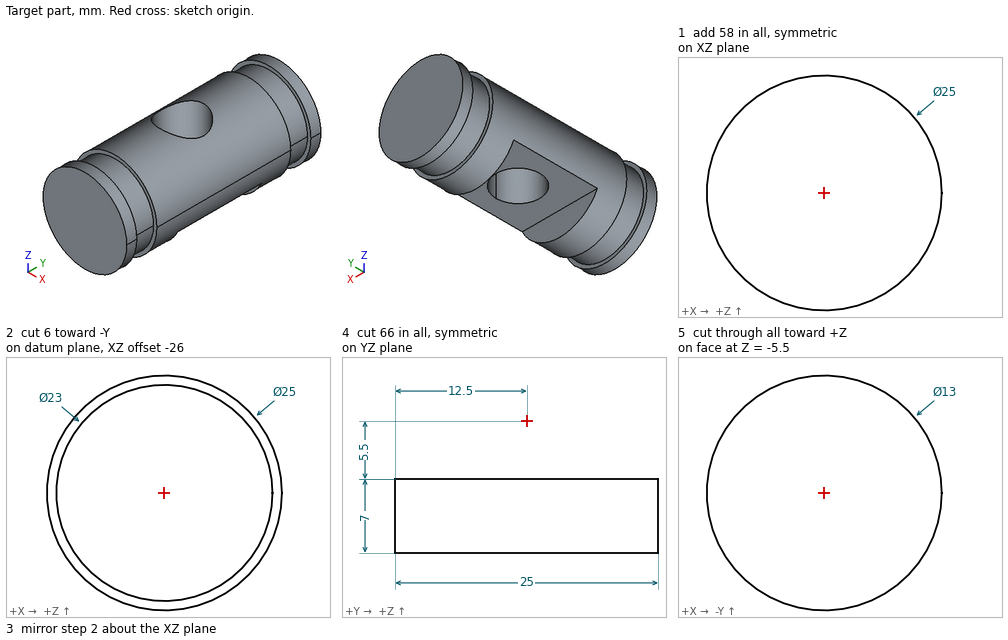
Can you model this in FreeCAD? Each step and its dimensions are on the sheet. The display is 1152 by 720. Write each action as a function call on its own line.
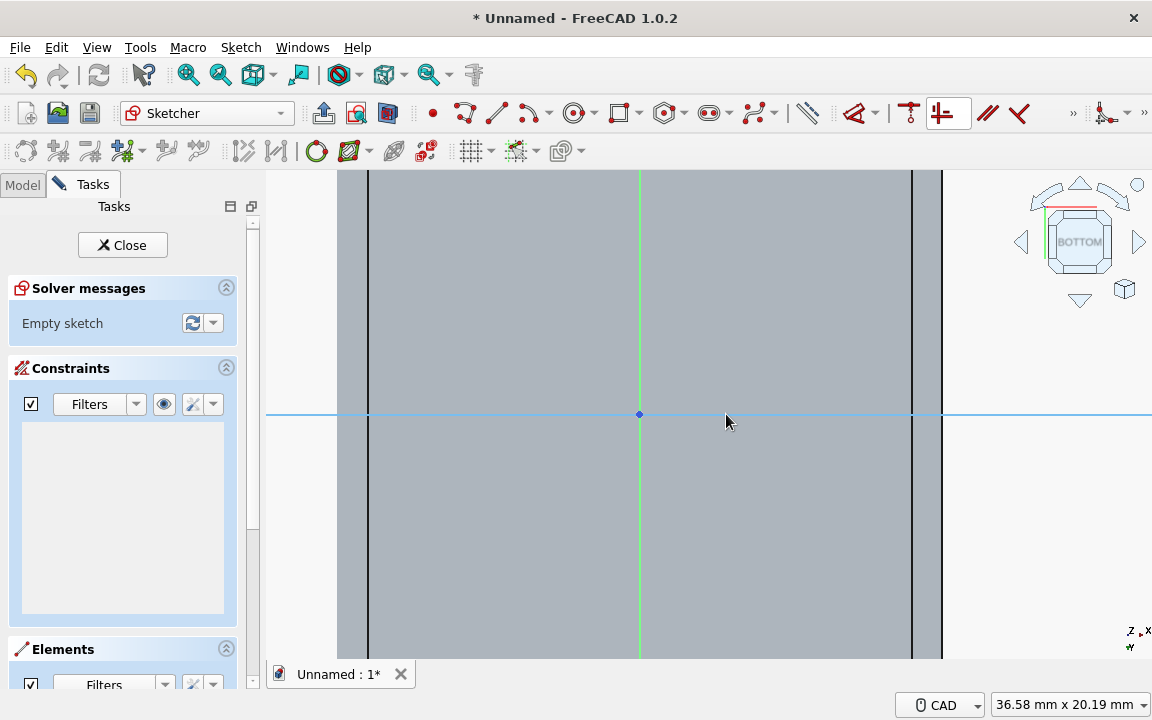
click(574, 114)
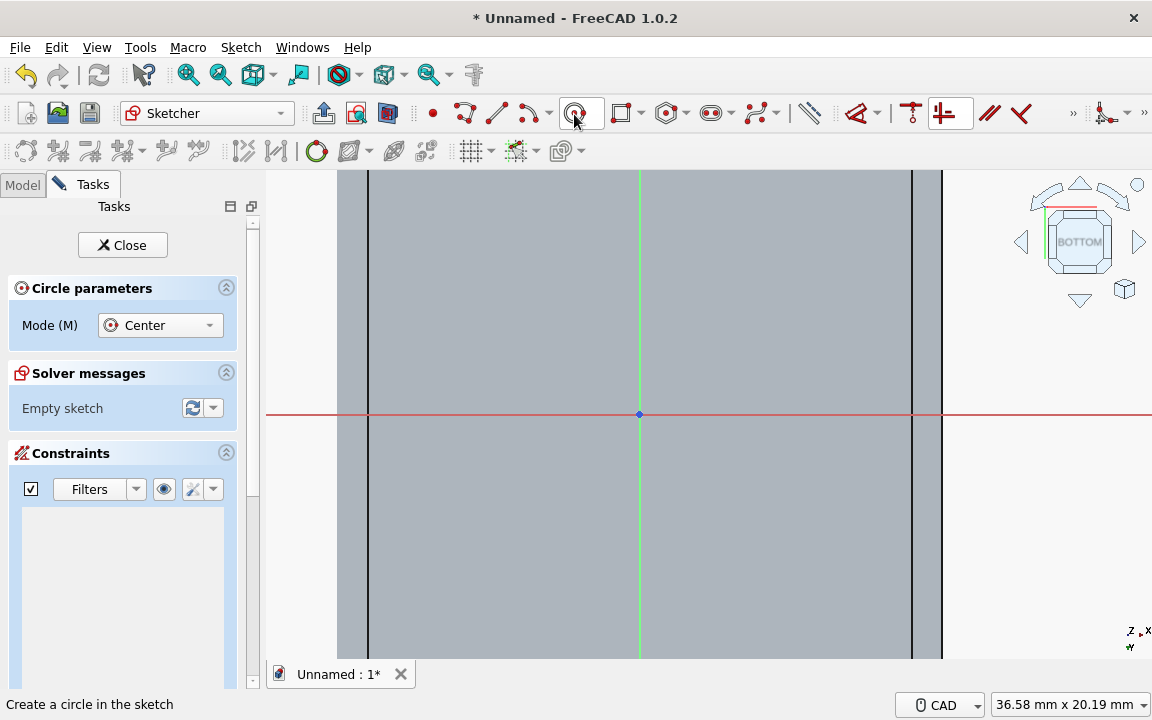
click(640, 414)
click(751, 303)
key(Escape)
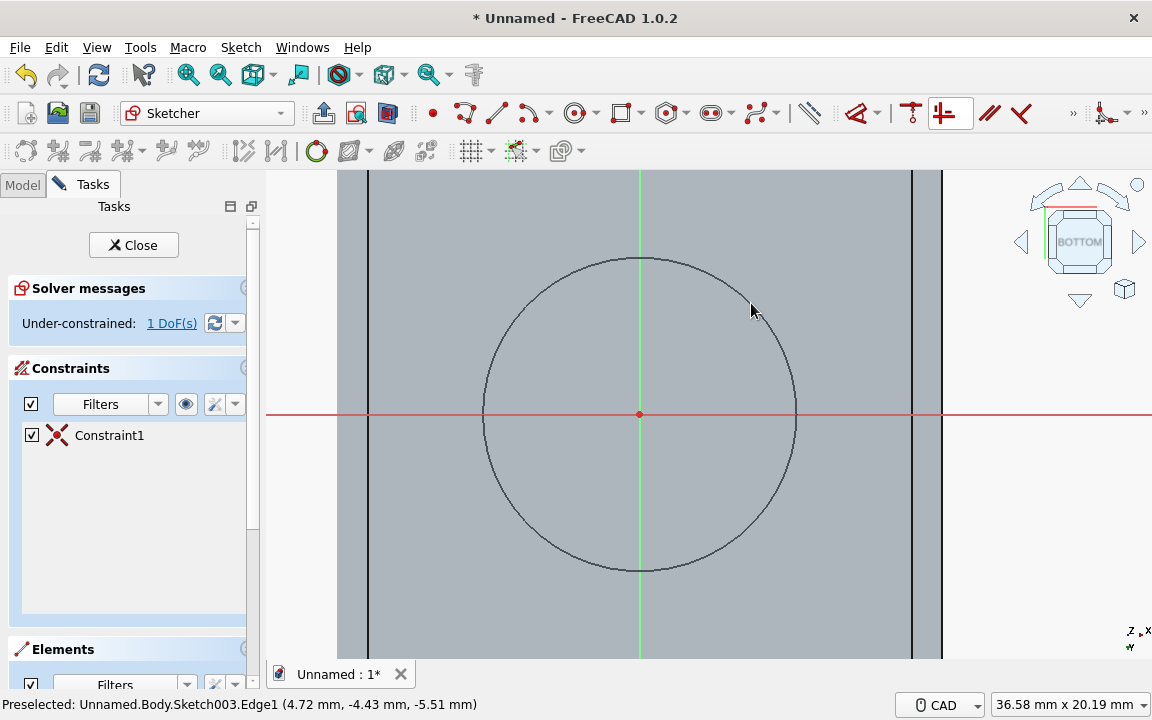
click(856, 114)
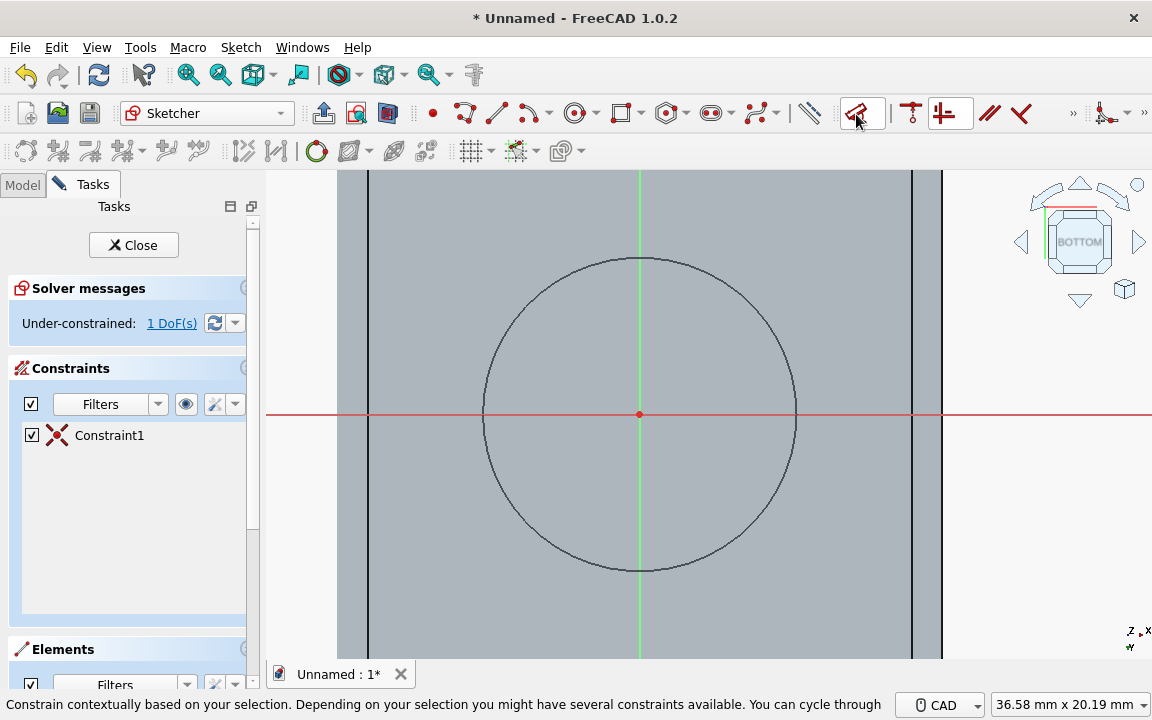
click(750, 303)
click(773, 280)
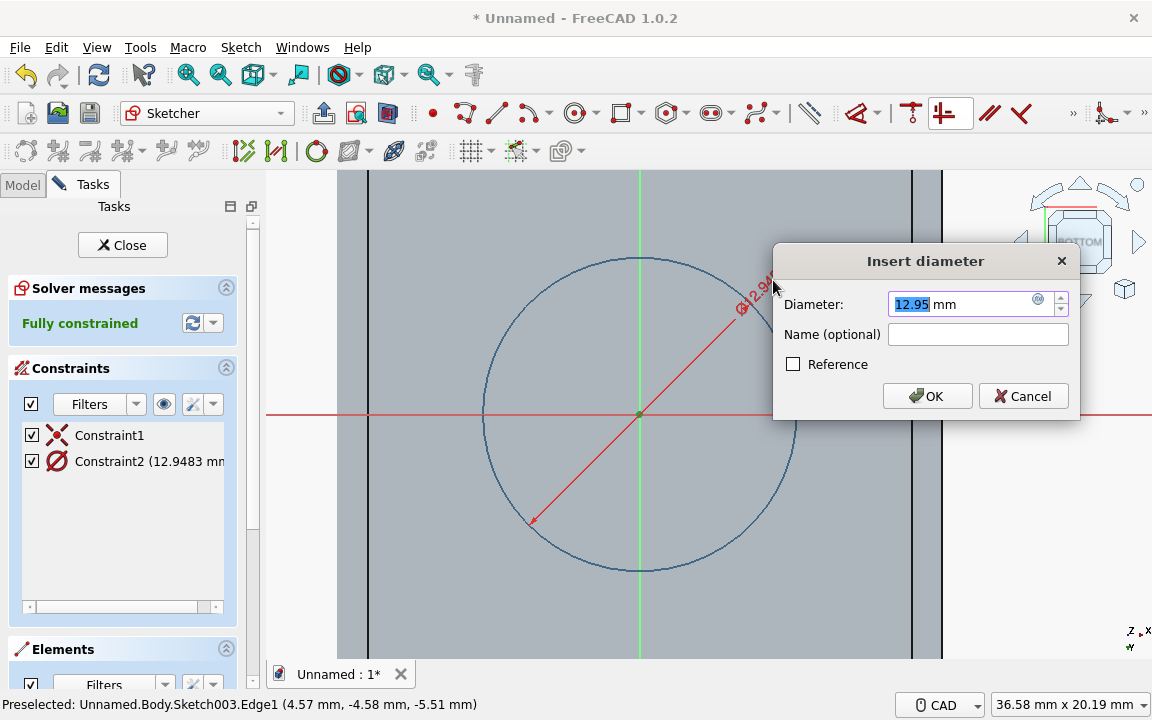
text(13)
key(Return)
key(Escape)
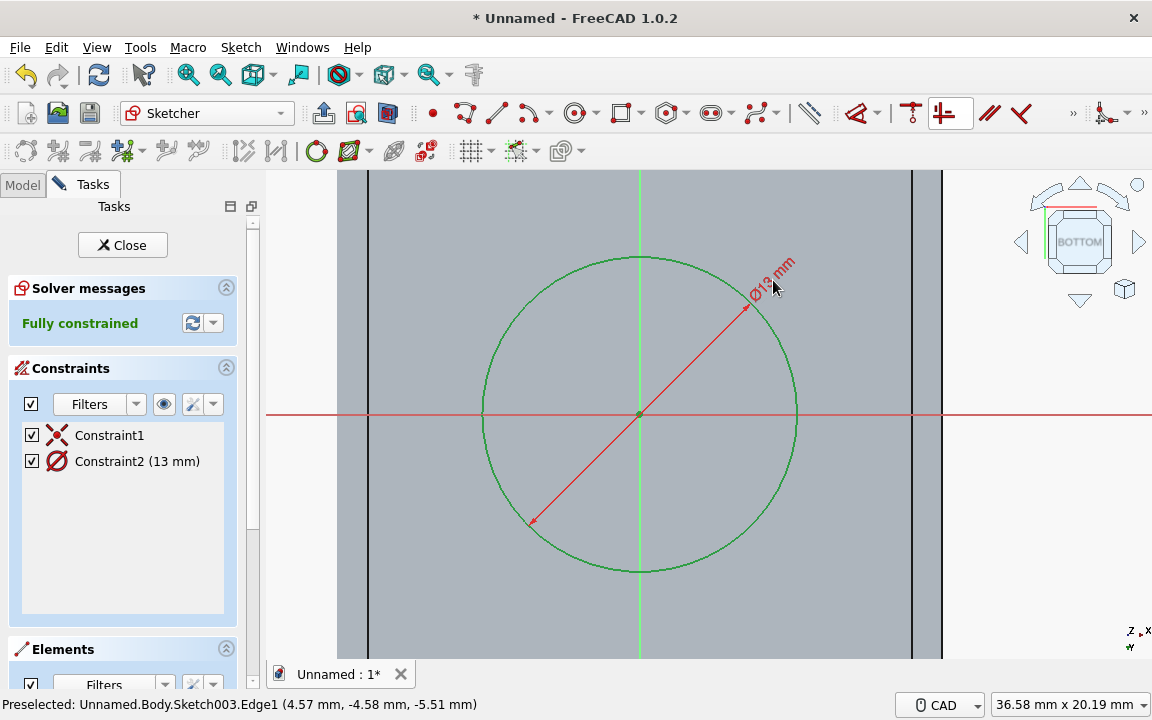
click(123, 245)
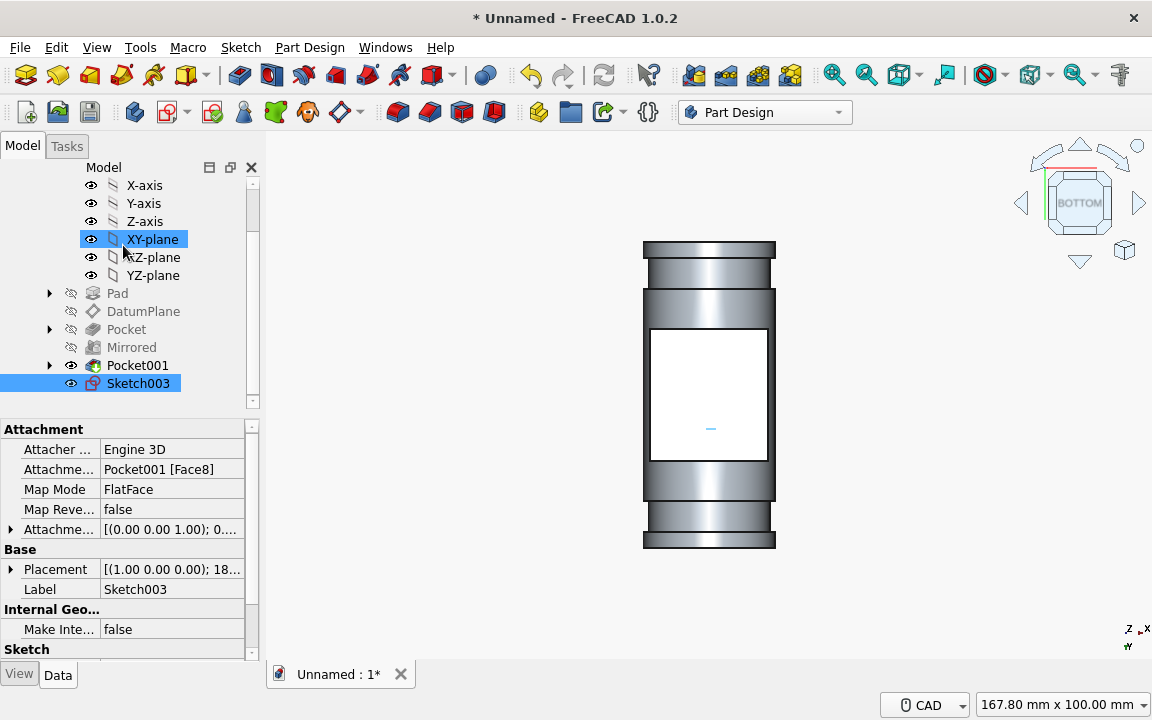
click(240, 76)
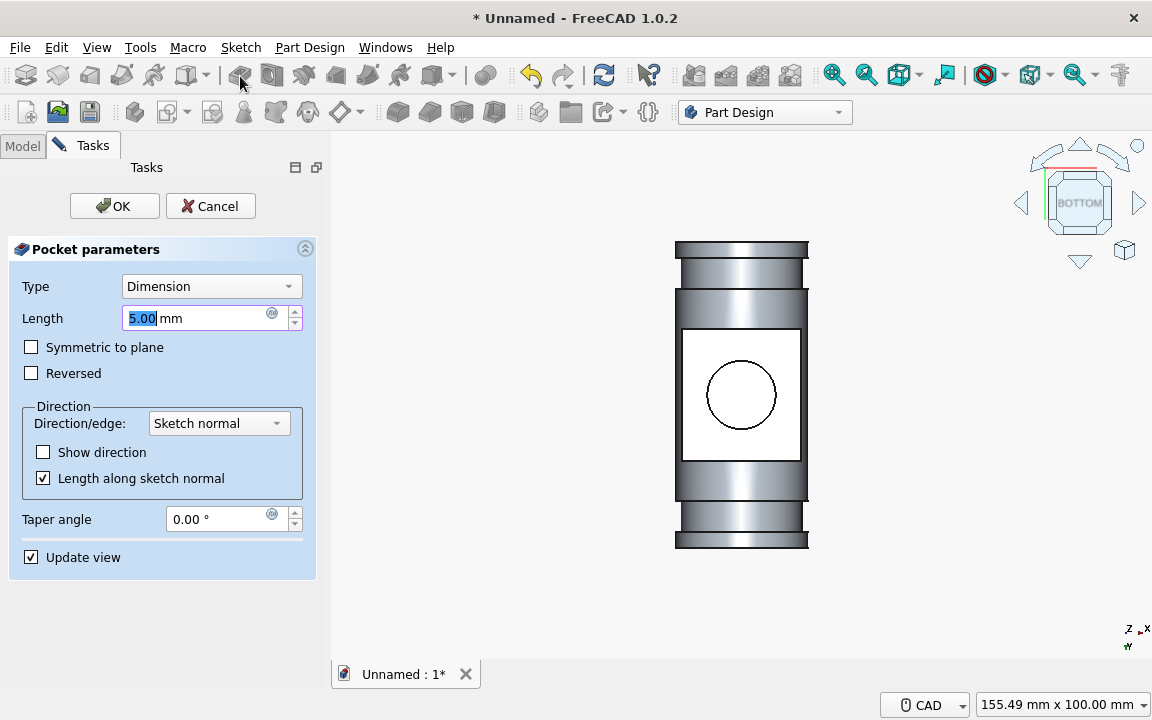
click(212, 286)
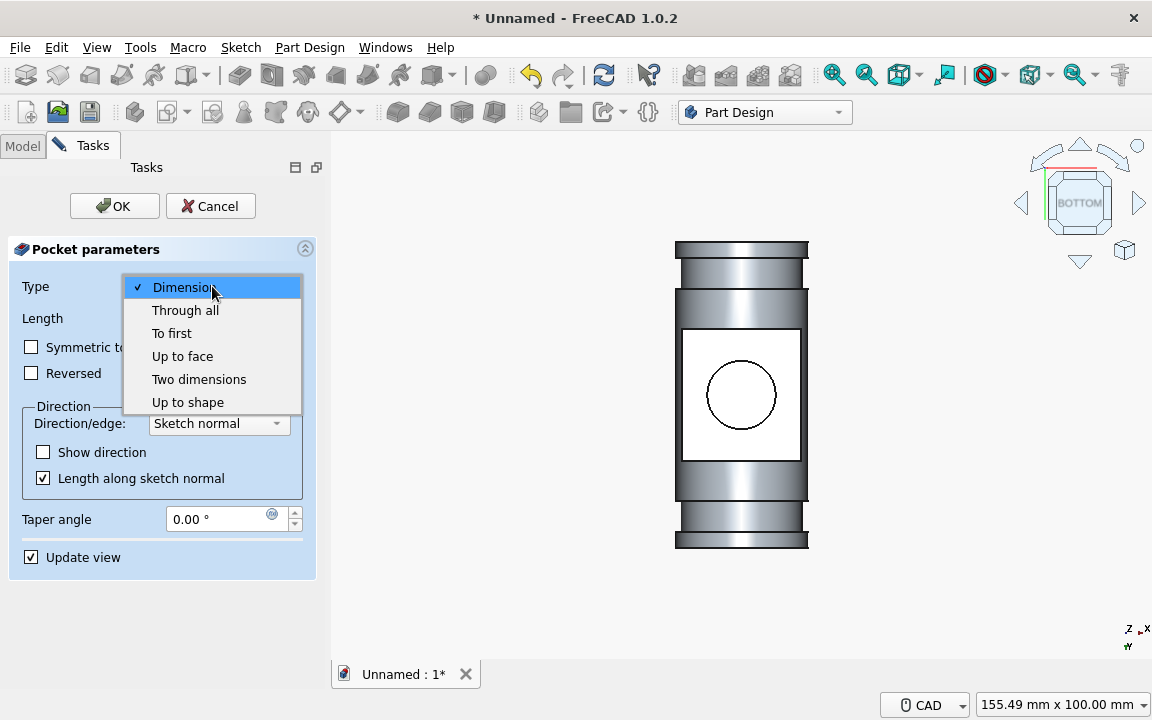
click(212, 310)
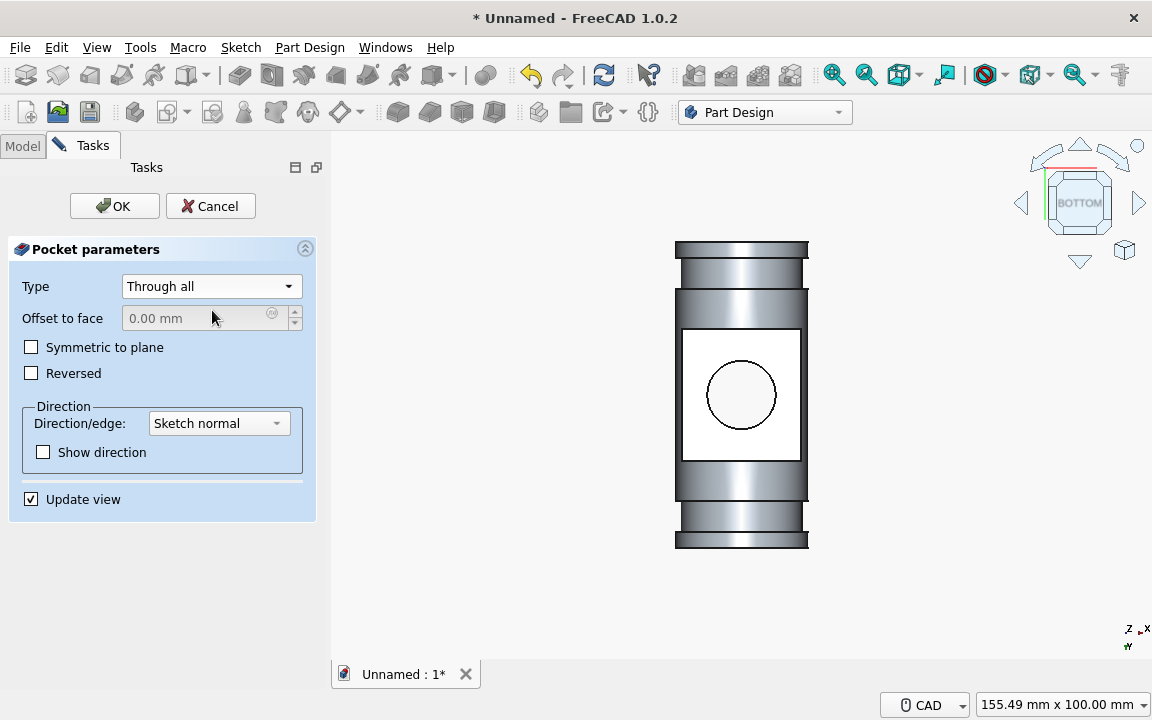
click(115, 206)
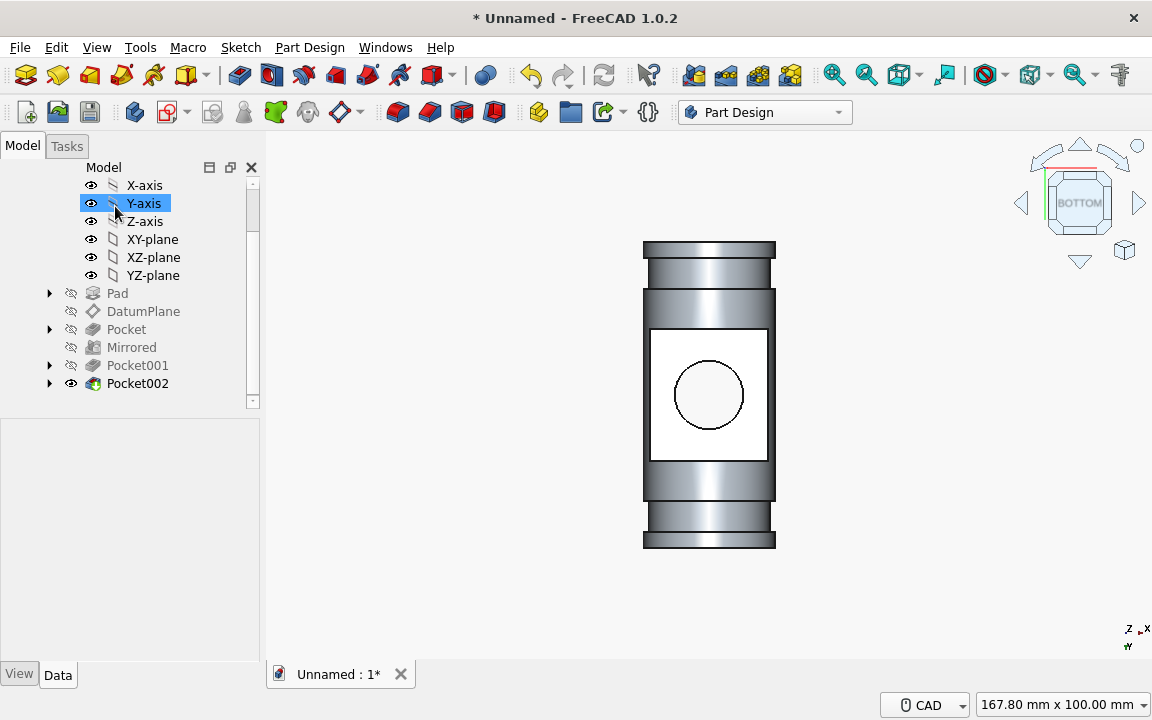
key(0)